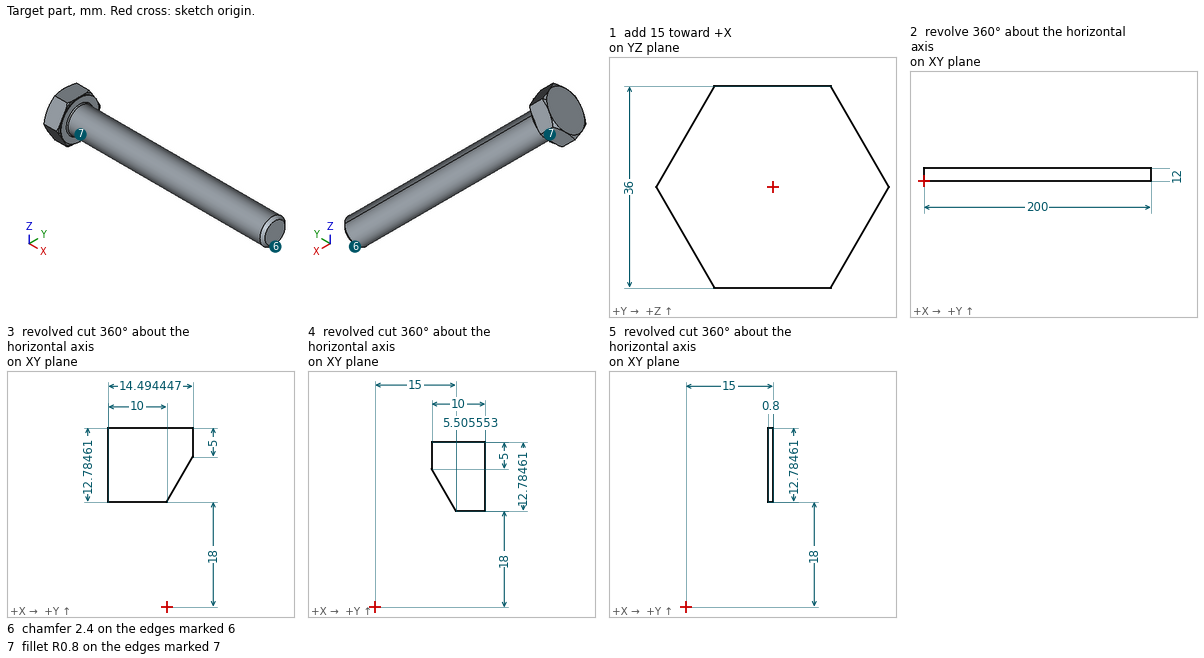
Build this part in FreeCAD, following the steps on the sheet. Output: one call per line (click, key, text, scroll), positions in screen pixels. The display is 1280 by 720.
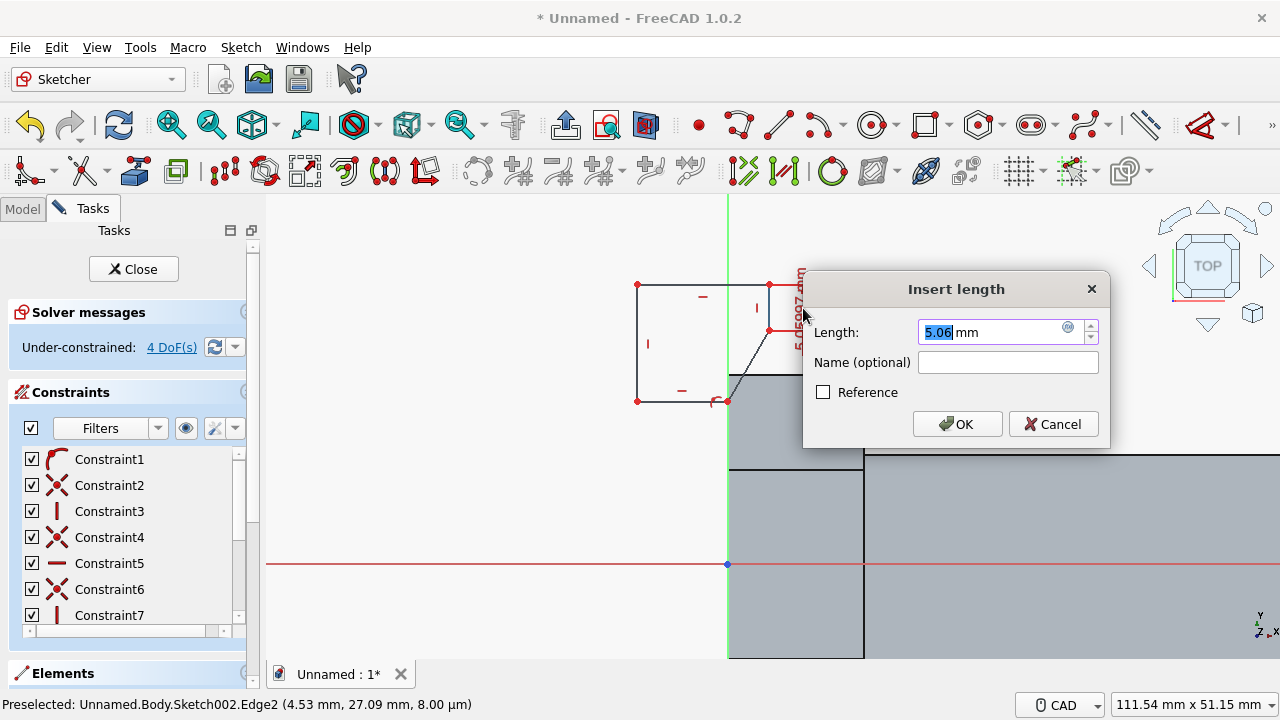
text(5)
key(Return)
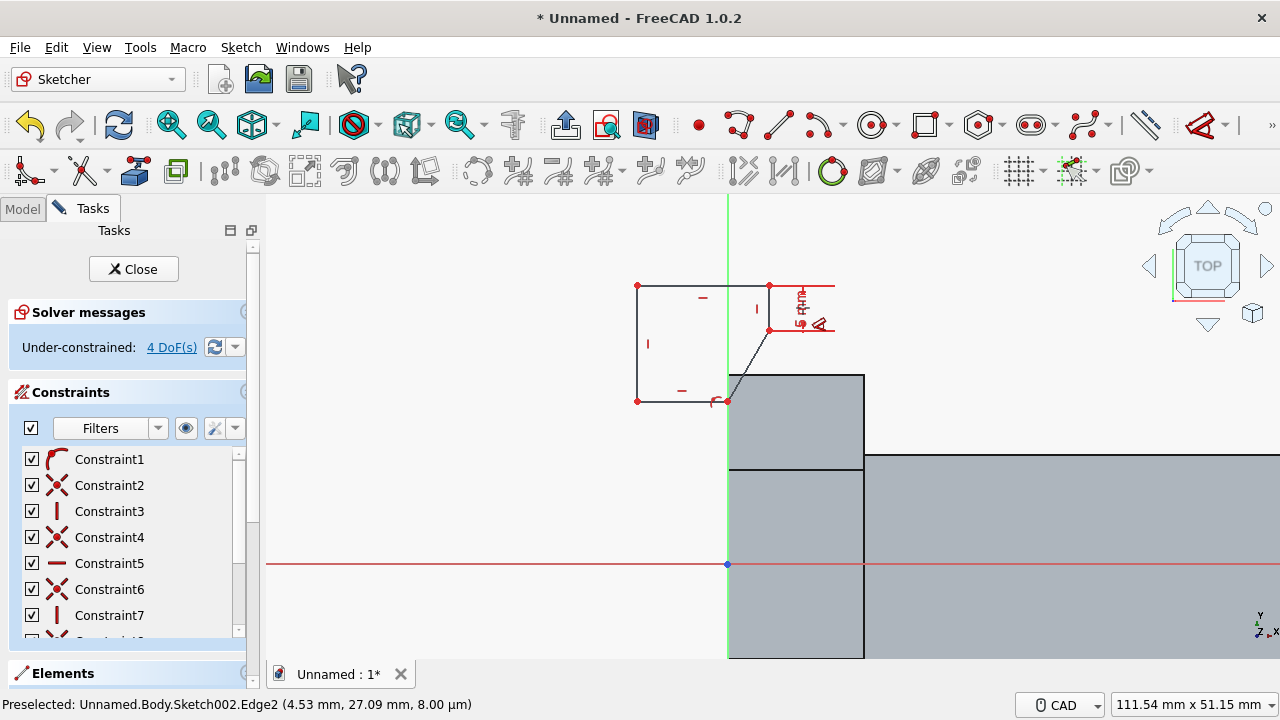
click(664, 402)
click(682, 368)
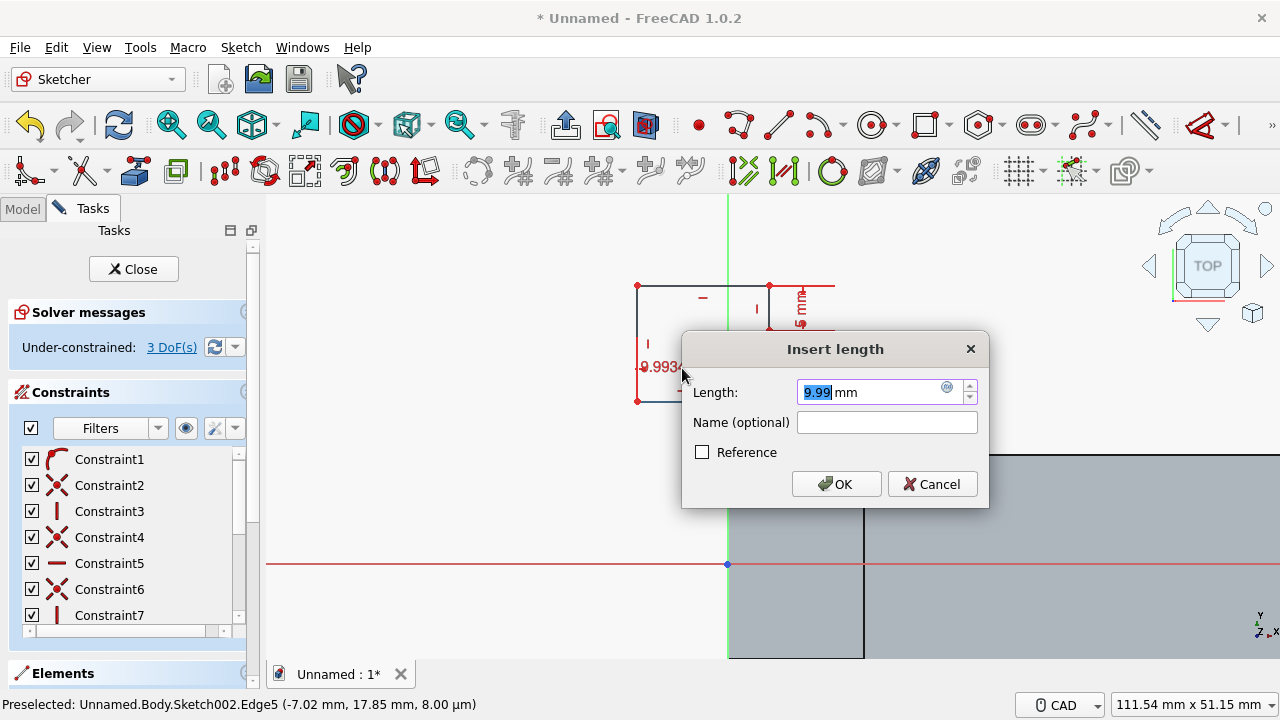
text(10)
key(Return)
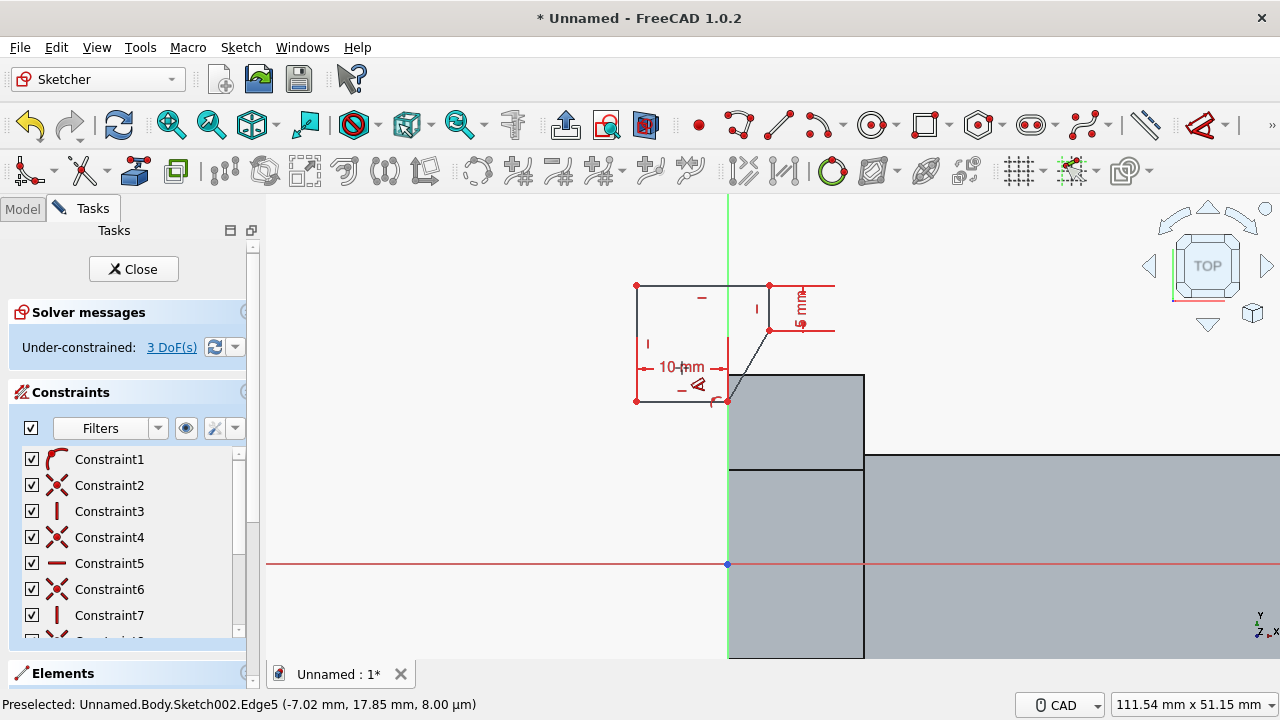
click(728, 402)
click(762, 483)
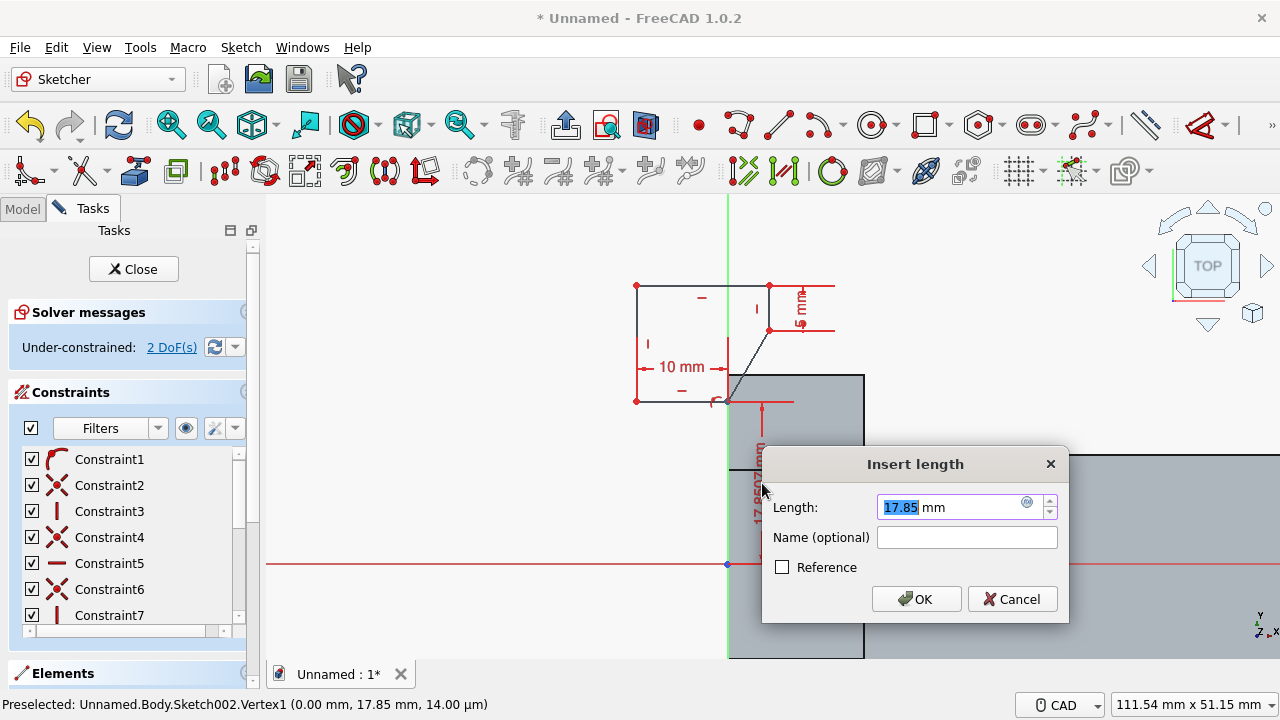
text(18)
key(Return)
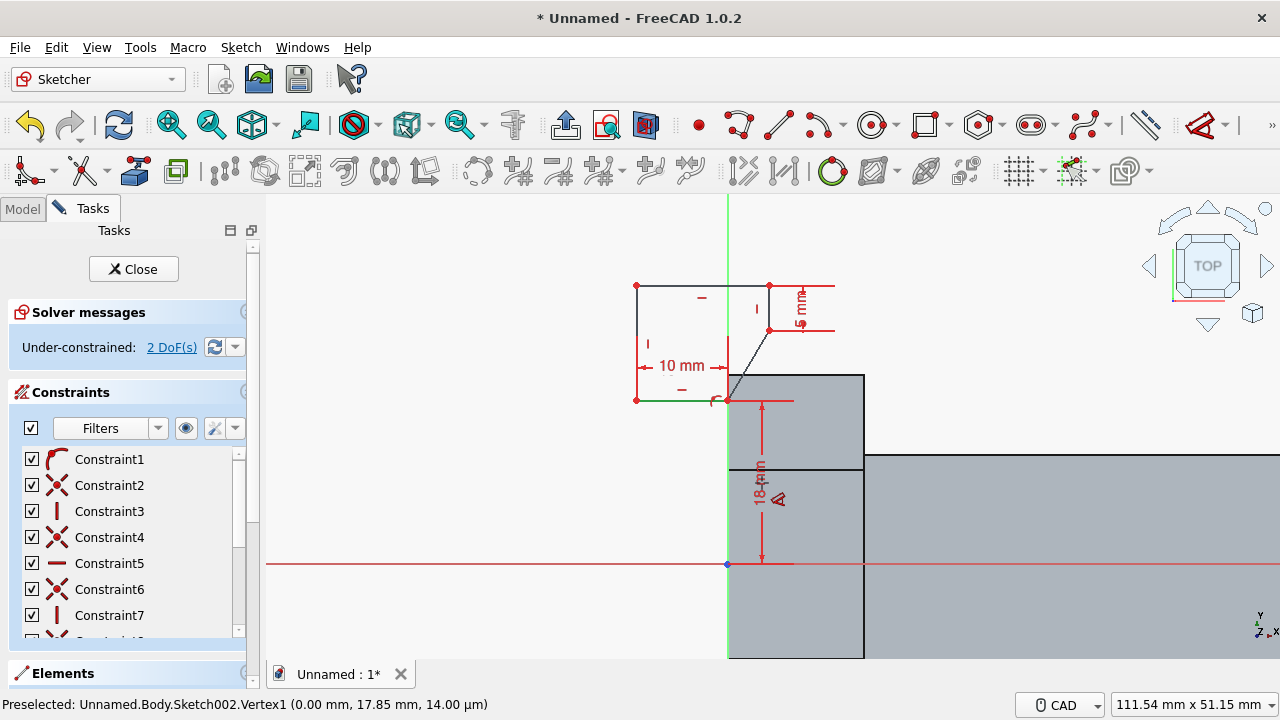
click(637, 320)
click(603, 343)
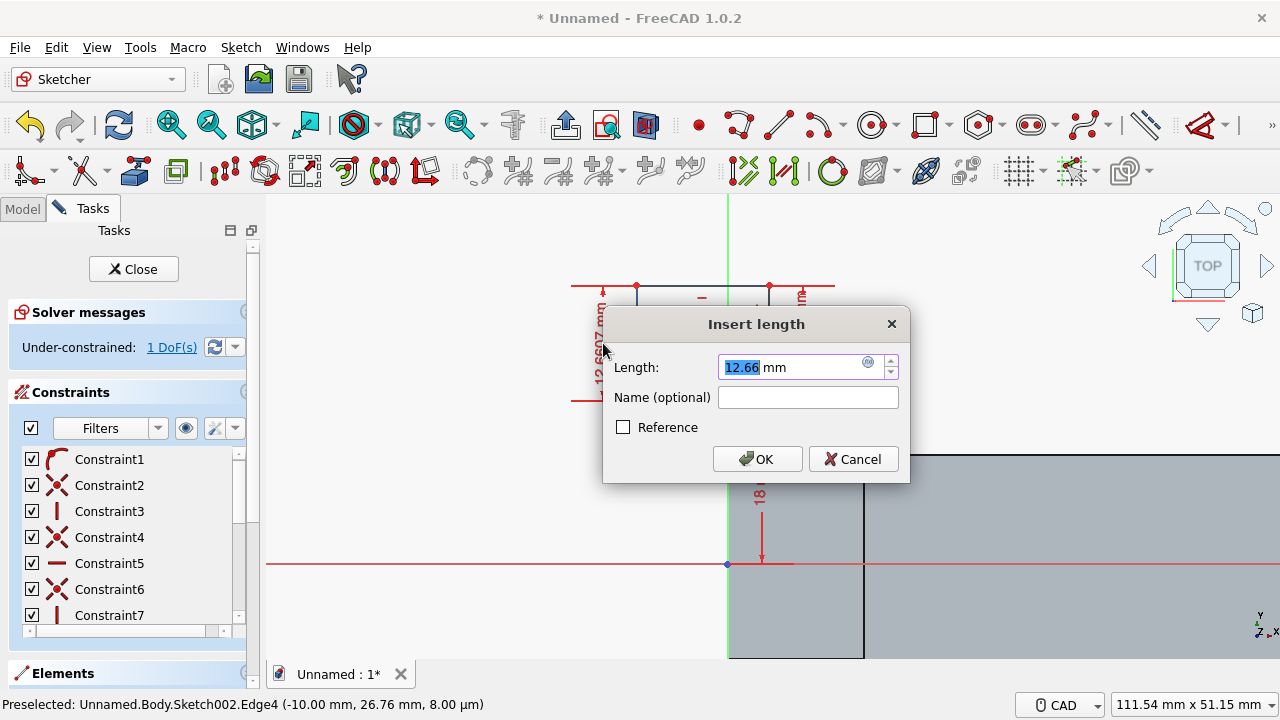
text(12.78461)
key(Return)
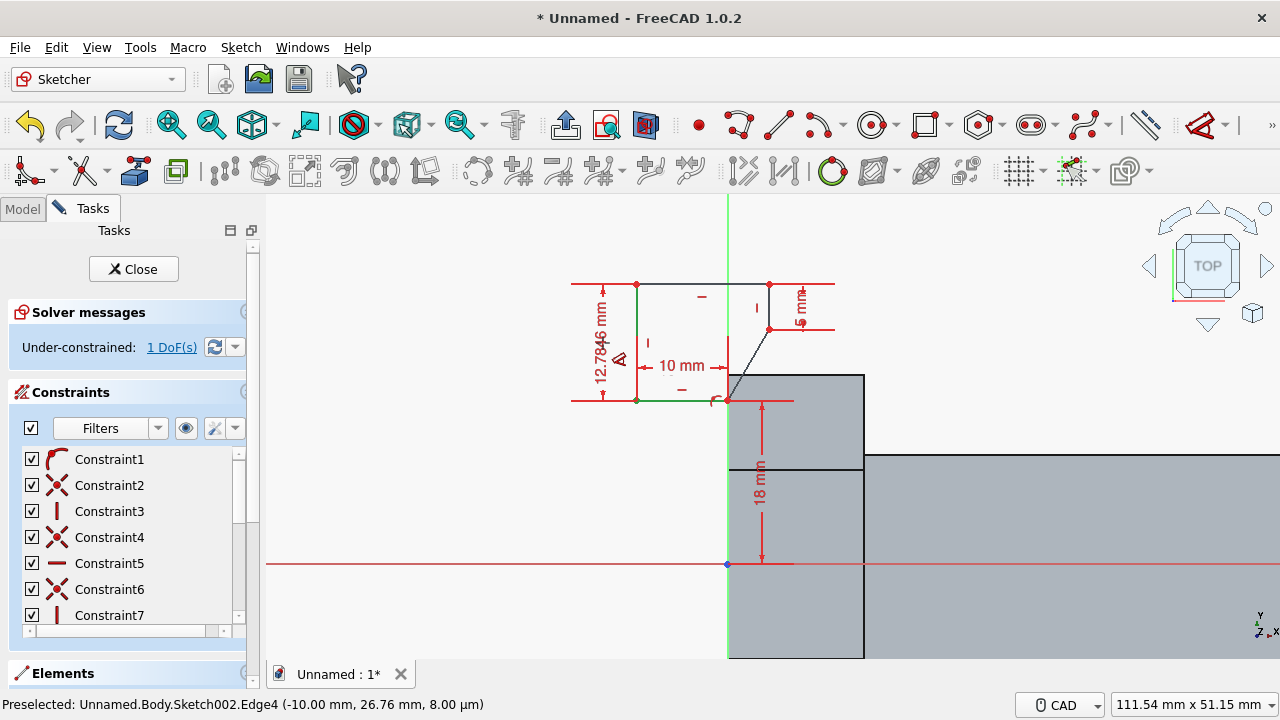
click(729, 284)
click(703, 250)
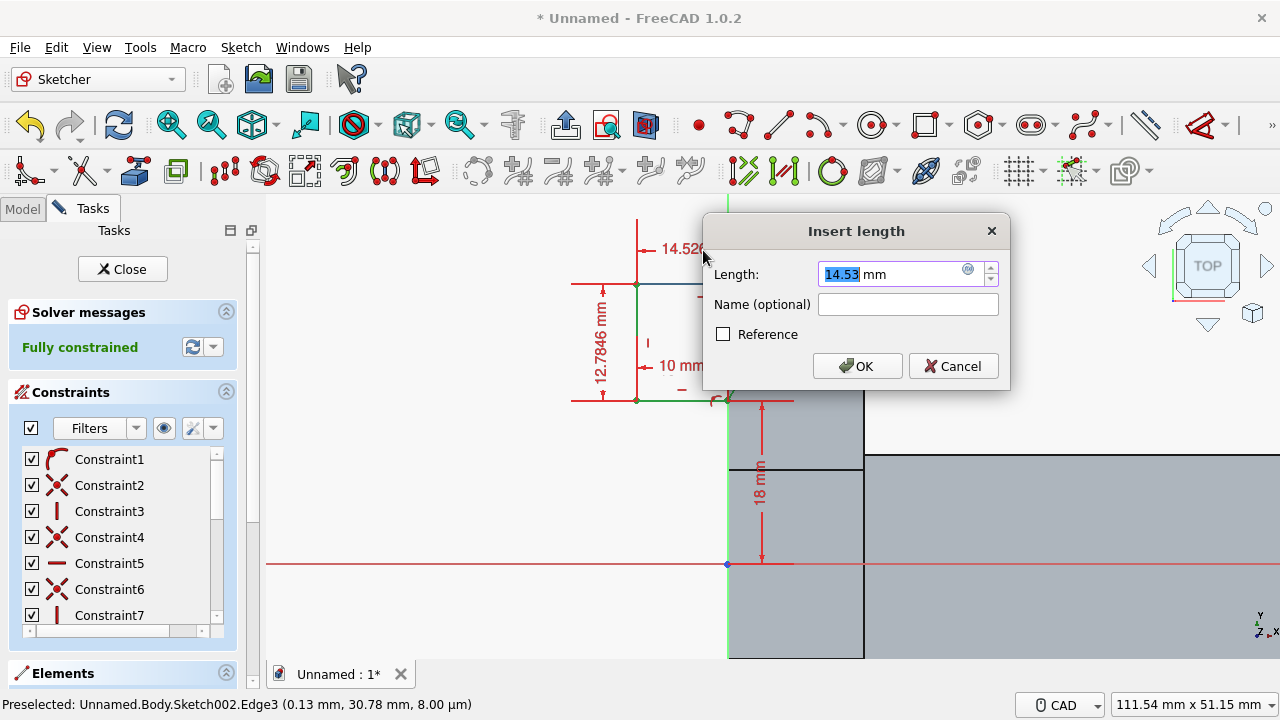
text(14.494447)
key(Return)
key(Escape)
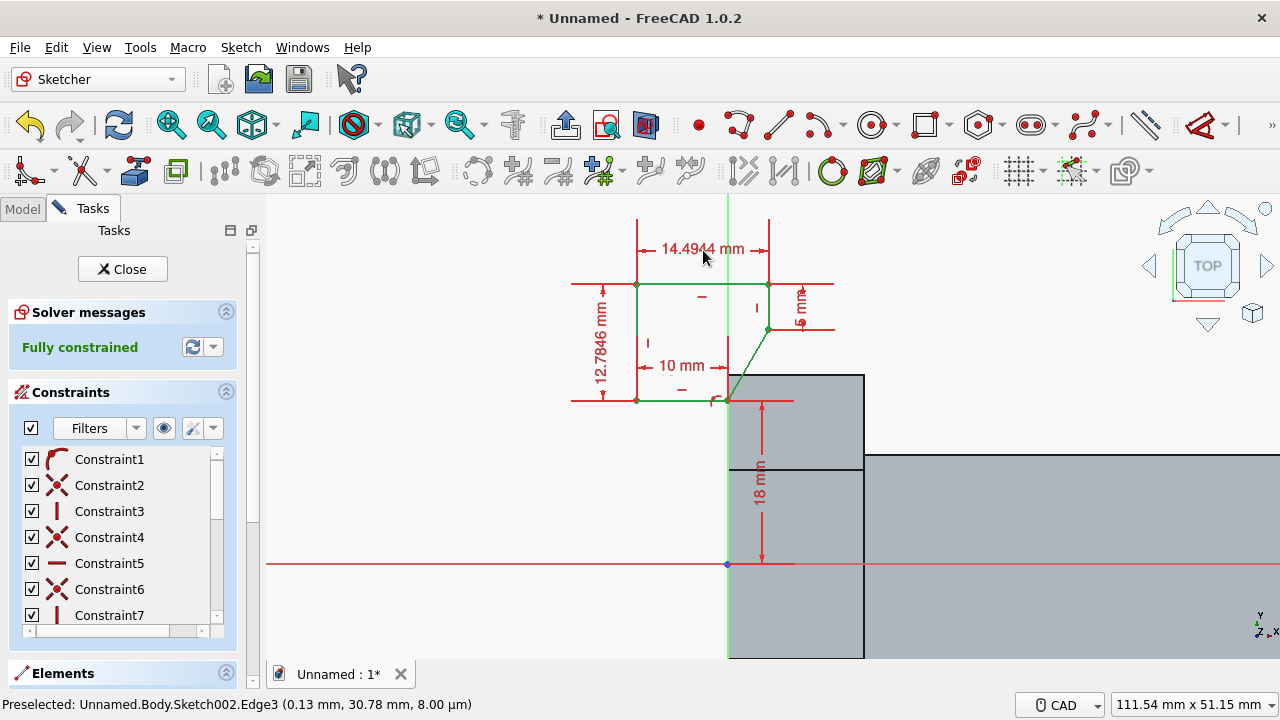
click(123, 269)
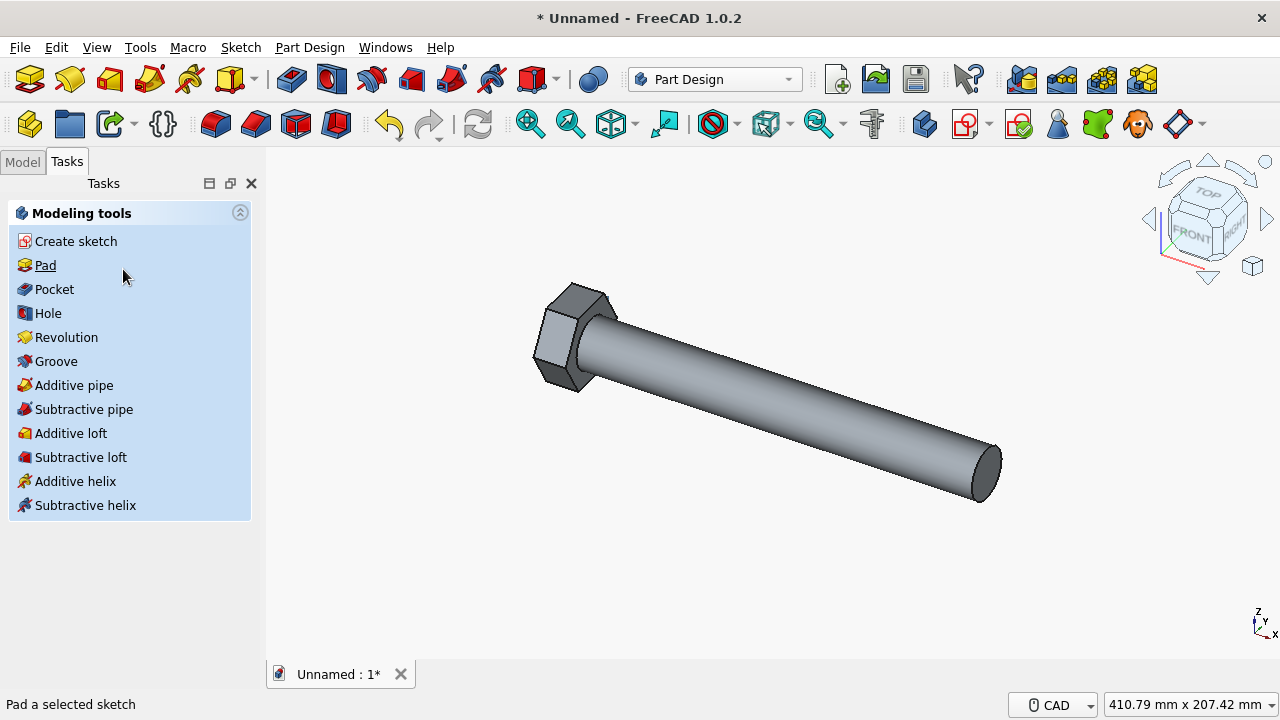
click(372, 80)